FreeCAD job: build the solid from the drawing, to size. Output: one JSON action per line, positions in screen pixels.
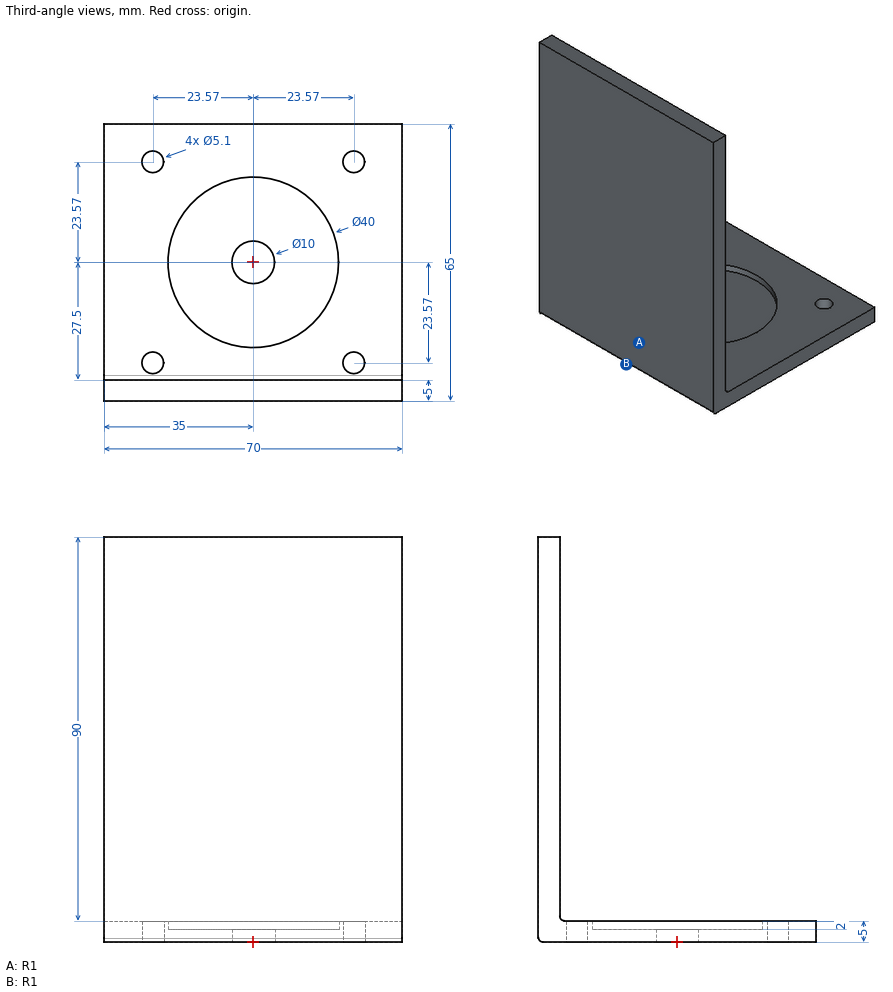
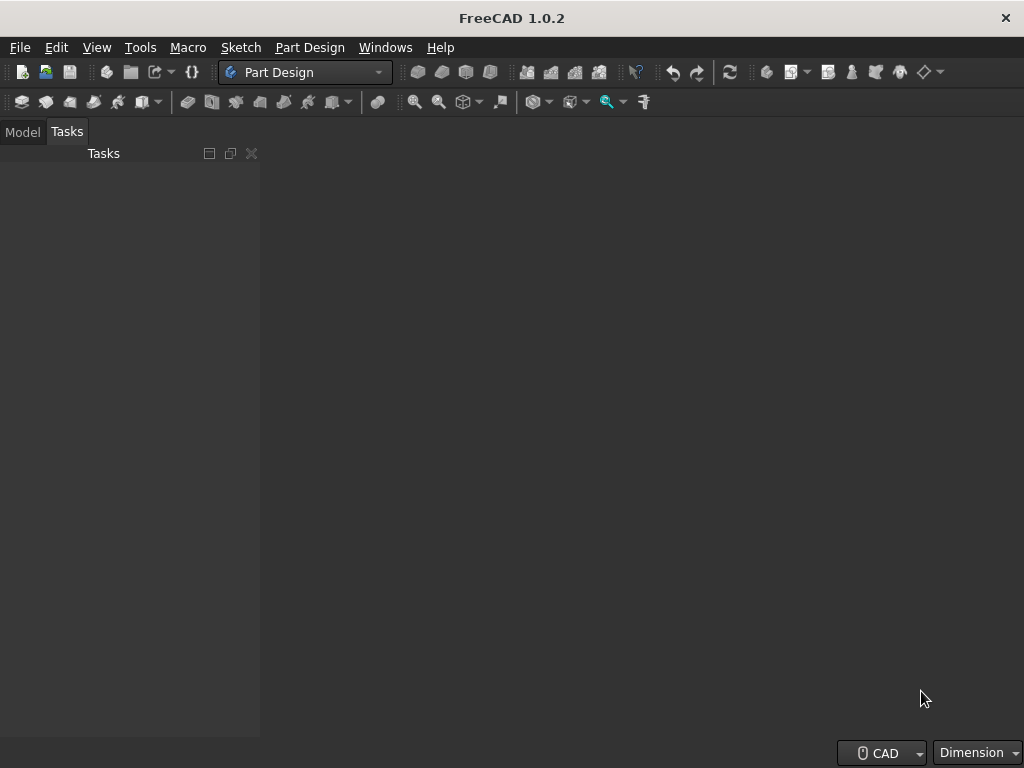
{"action": "left_click", "coordinate": [22, 72]}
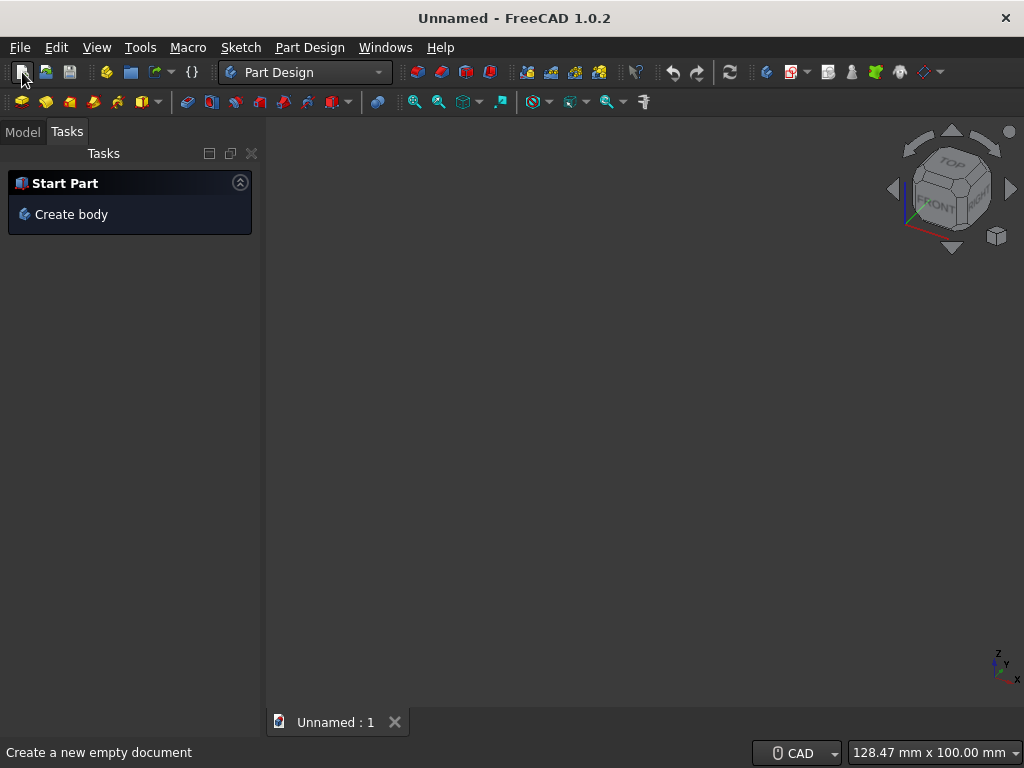
{"action": "left_click", "coordinate": [792, 72]}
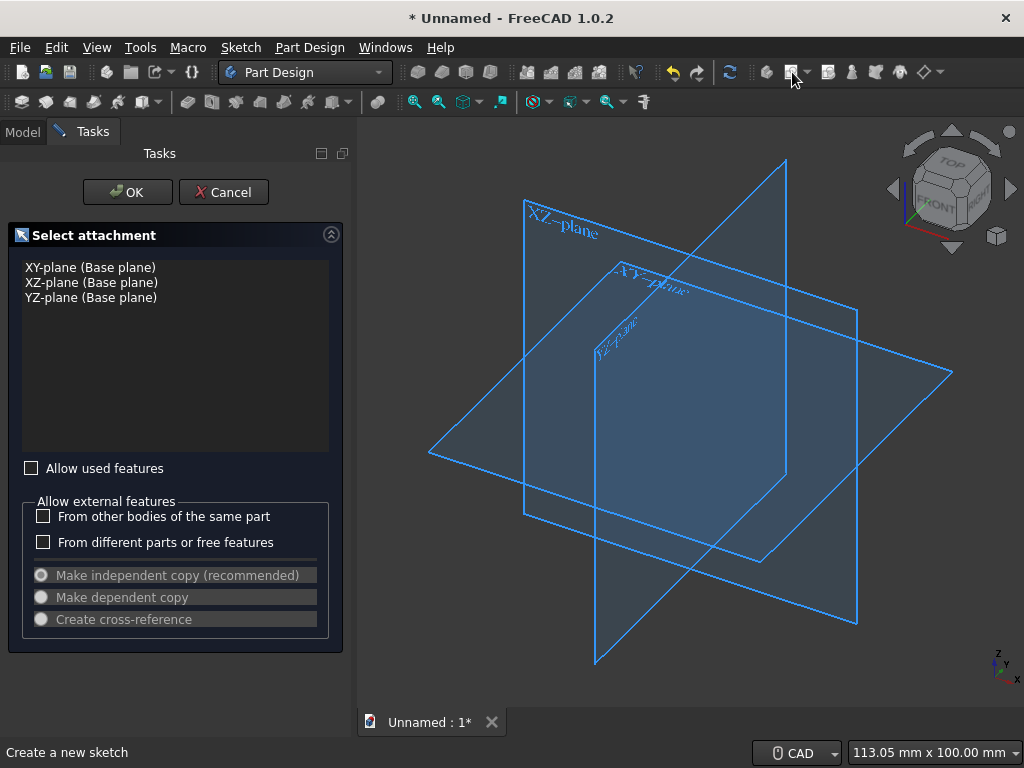
{"action": "left_click", "coordinate": [82, 268]}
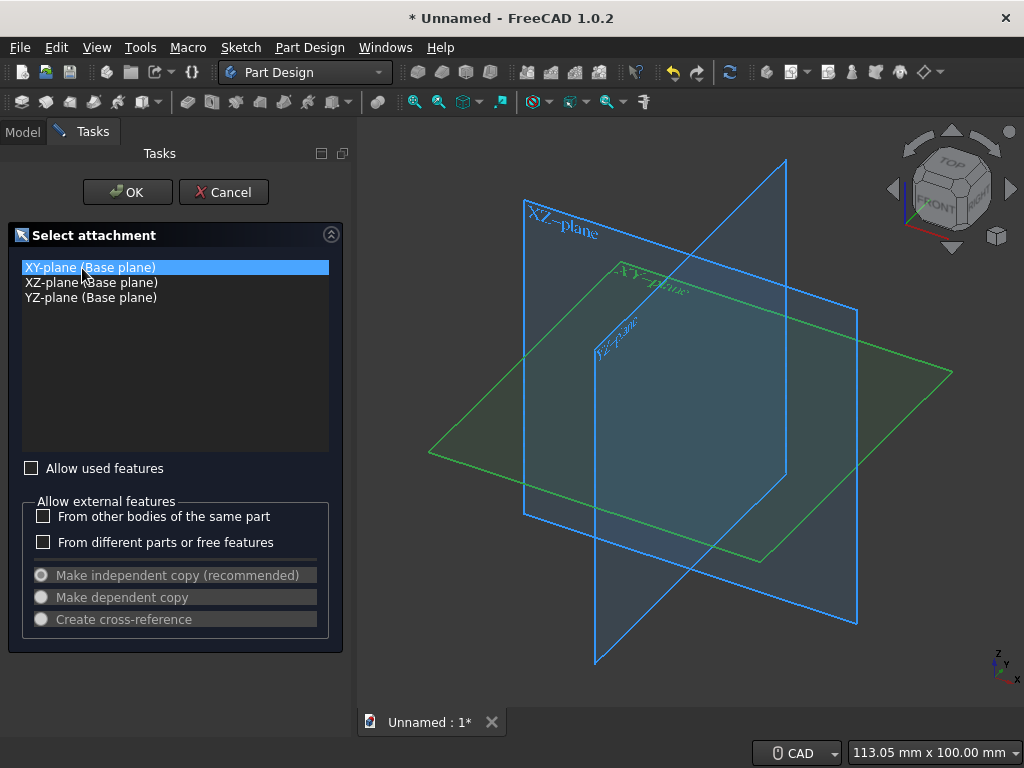
{"action": "left_click", "coordinate": [128, 192]}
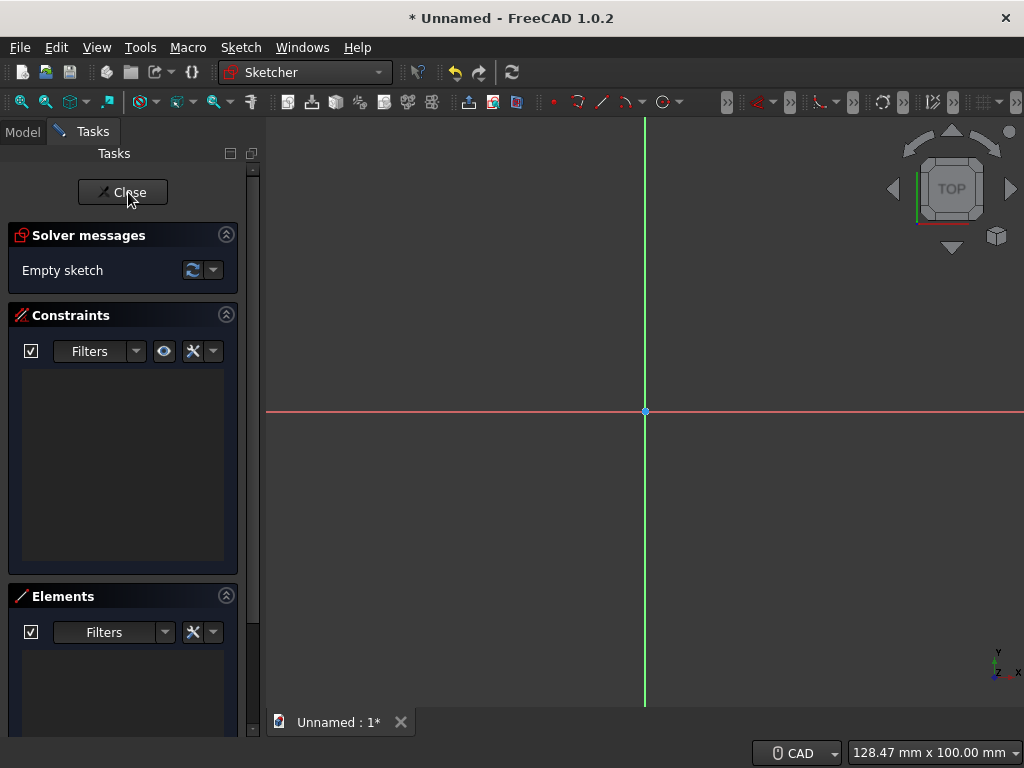
{"action": "scroll", "coordinate": [294, 412], "scroll_direction": "down", "scroll_amount": 1}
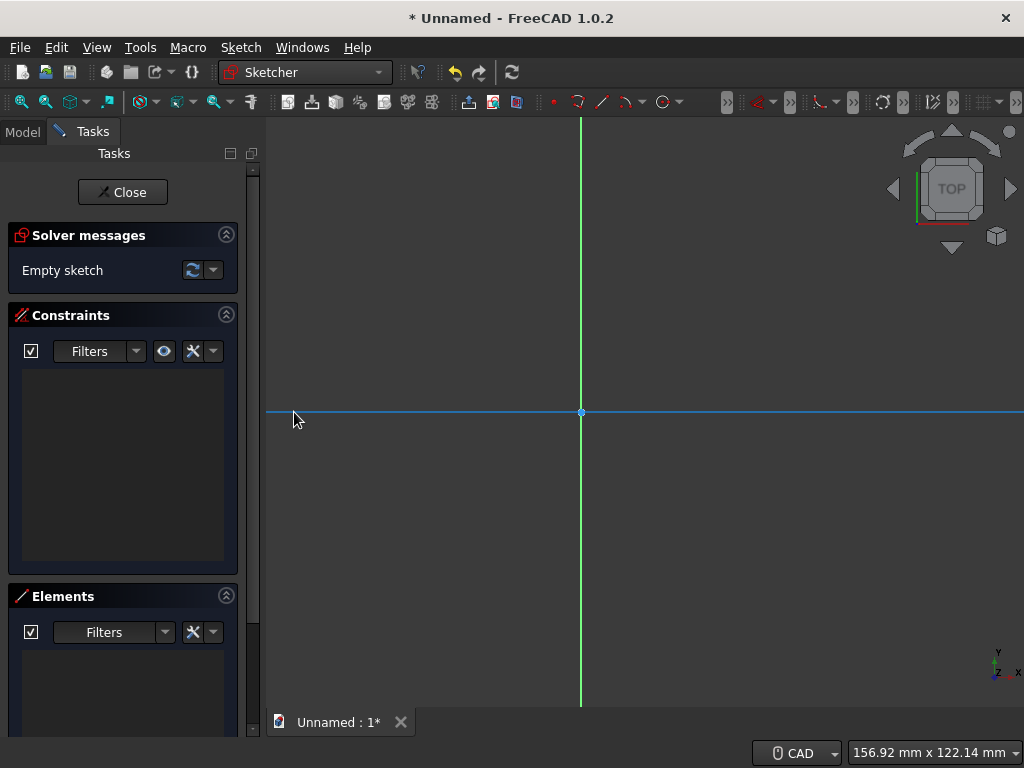
{"action": "key", "text": "g v"}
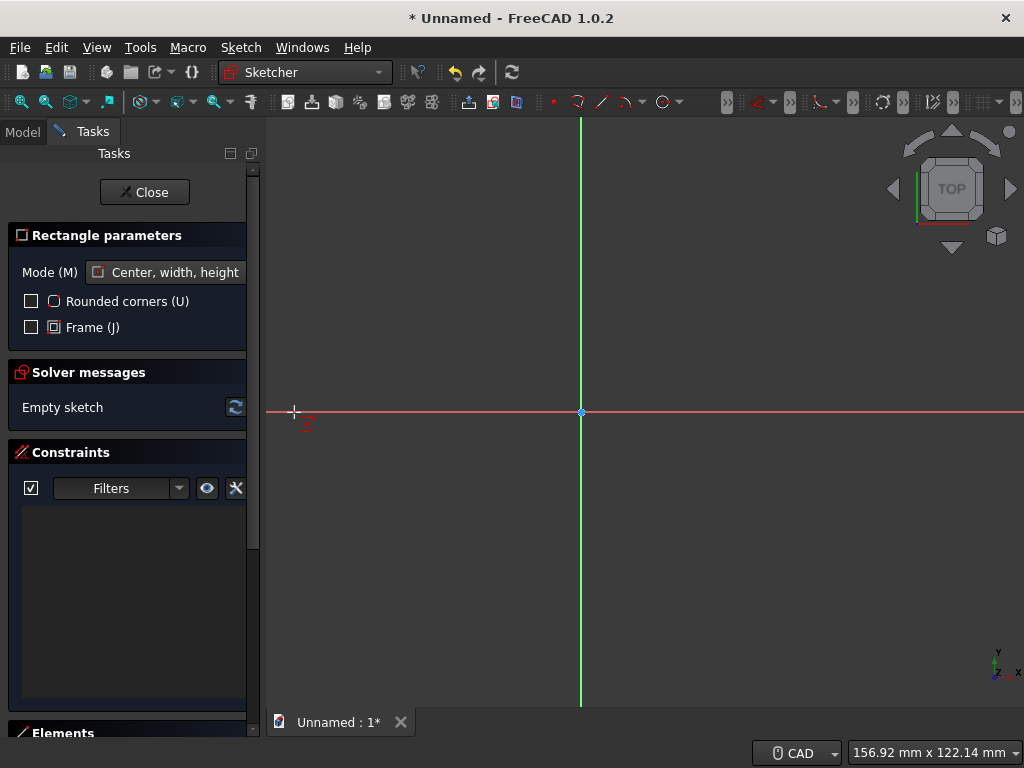
{"action": "left_click", "coordinate": [581, 412]}
{"action": "mouse_move", "coordinate": [750, 255]}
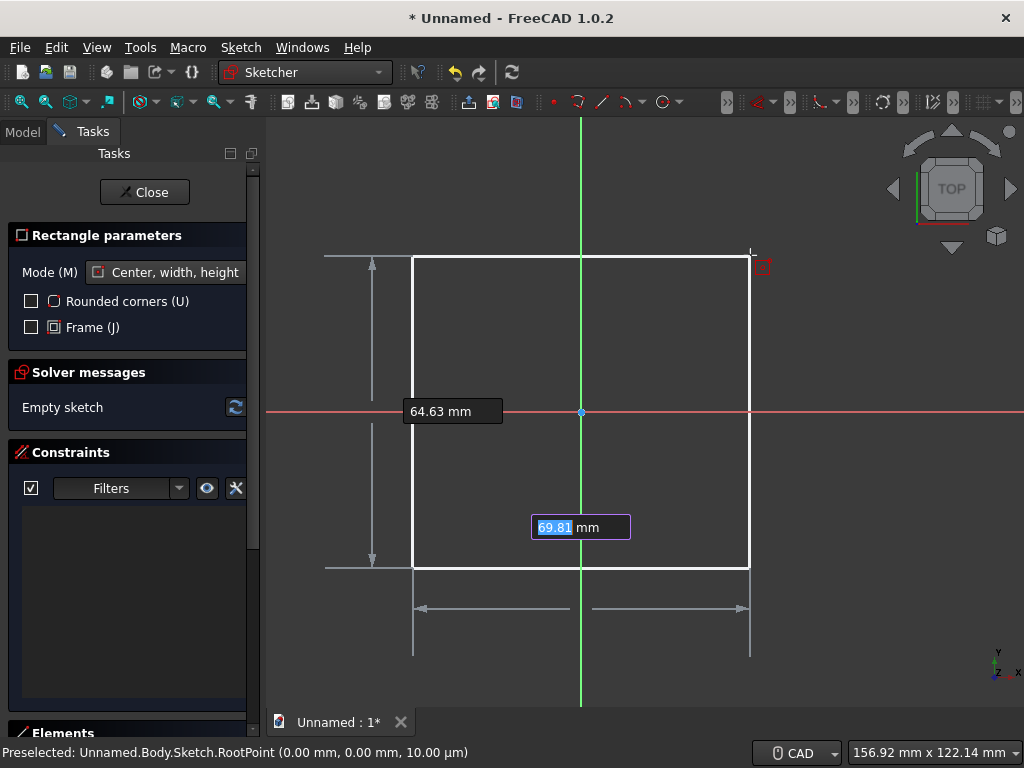
{"action": "type", "text": "70"}
{"action": "key", "text": "Tab"}
{"action": "type", "text": "65"}
{"action": "key", "text": "Return"}
{"action": "key", "text": "Escape"}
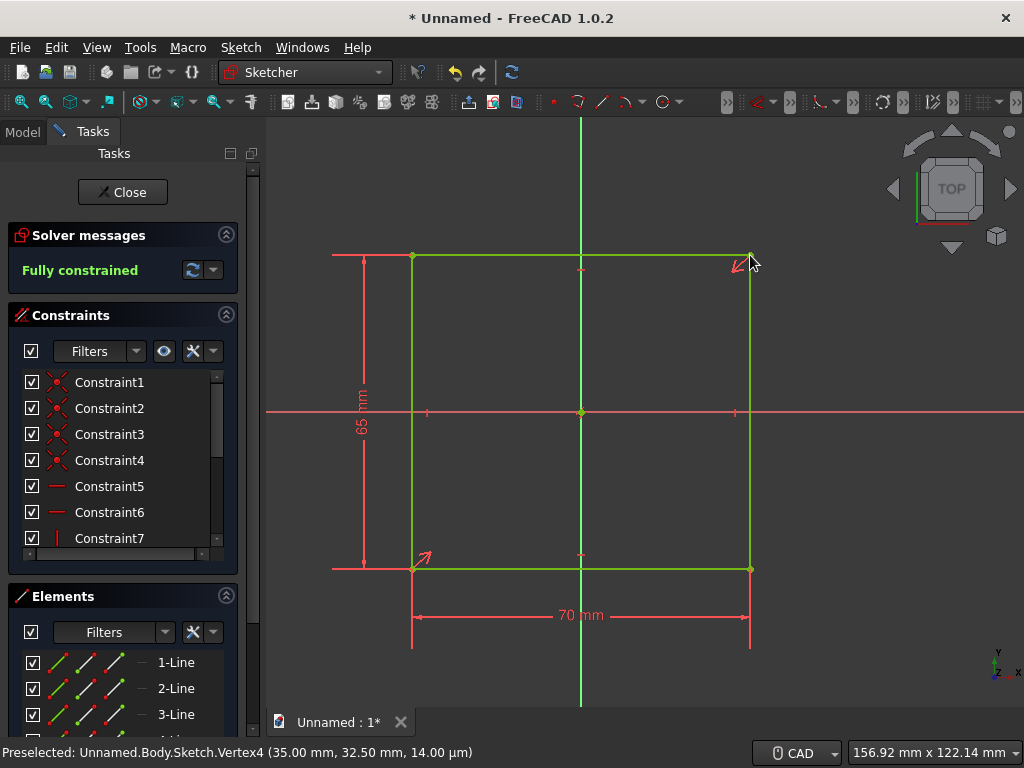
{"action": "left_click", "coordinate": [123, 192]}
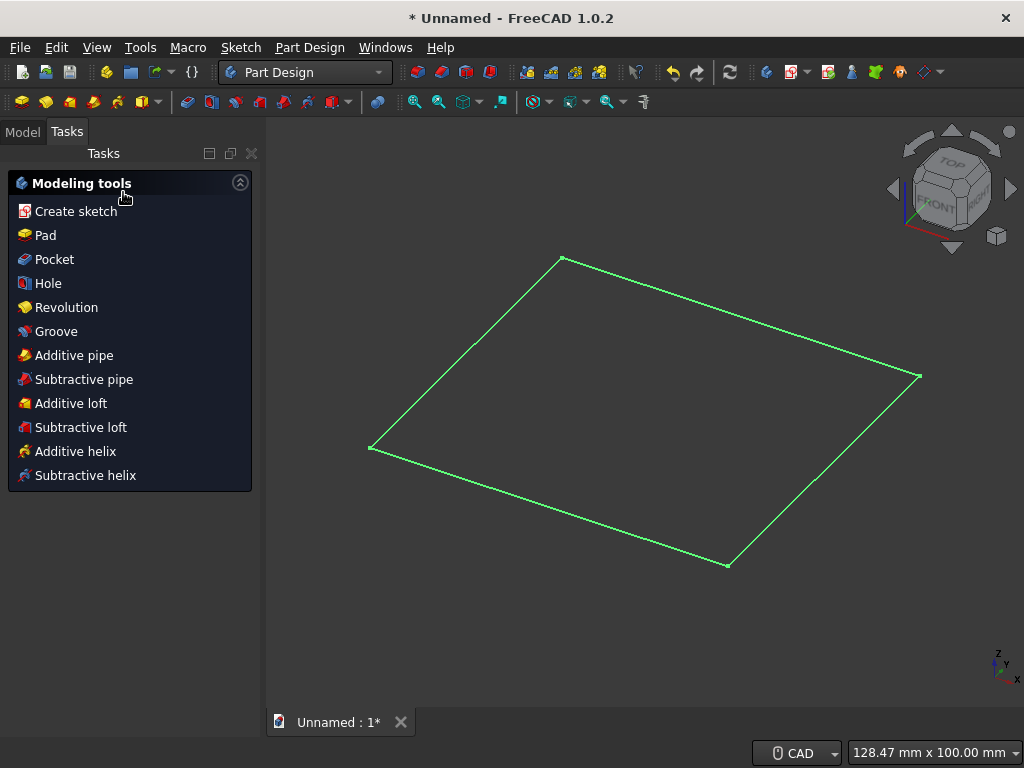
{"action": "left_click", "coordinate": [22, 102]}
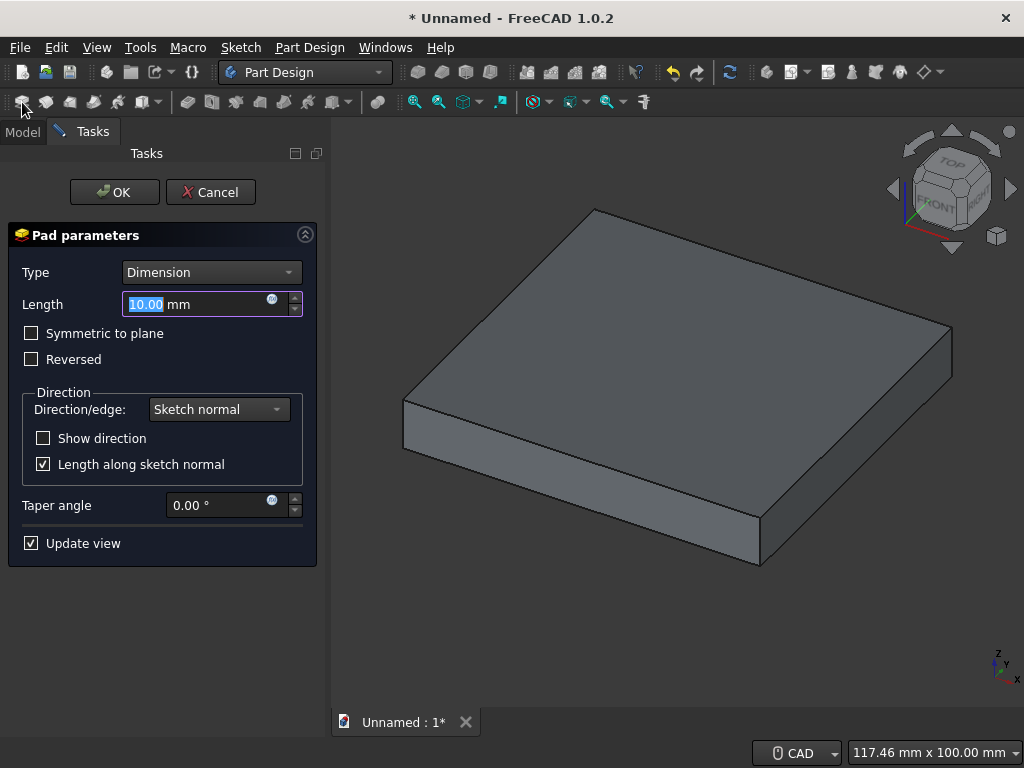
{"action": "type", "text": "5"}
{"action": "key", "text": "Tab"}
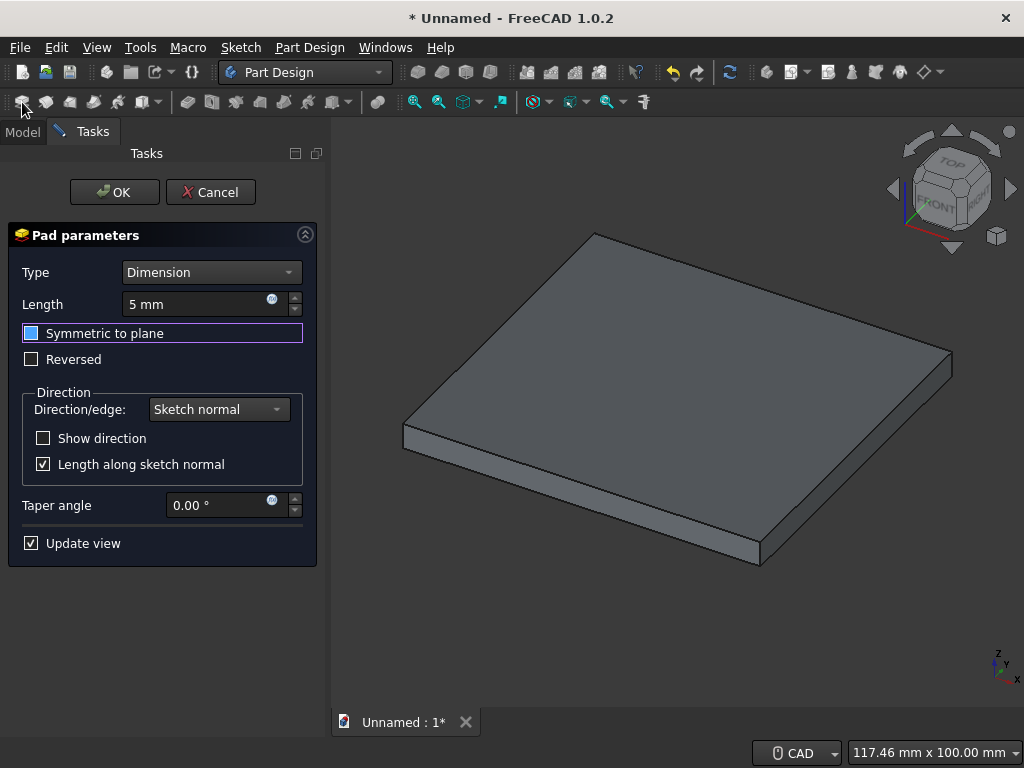
{"action": "left_click", "coordinate": [115, 192]}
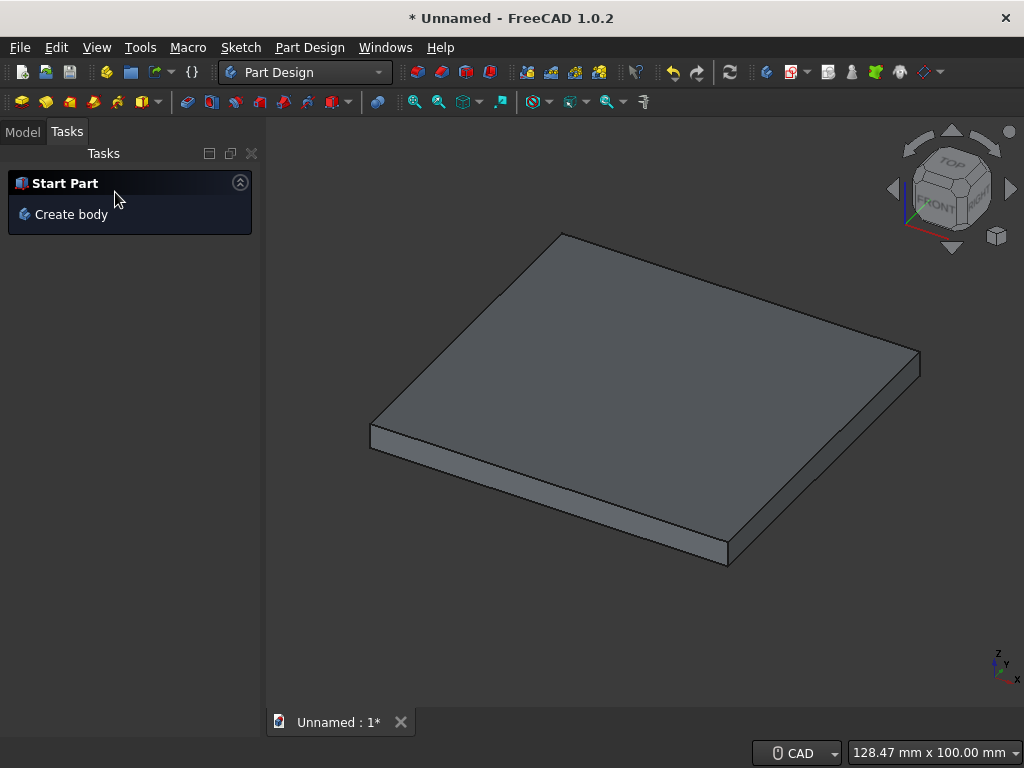
{"action": "left_click", "coordinate": [645, 387]}